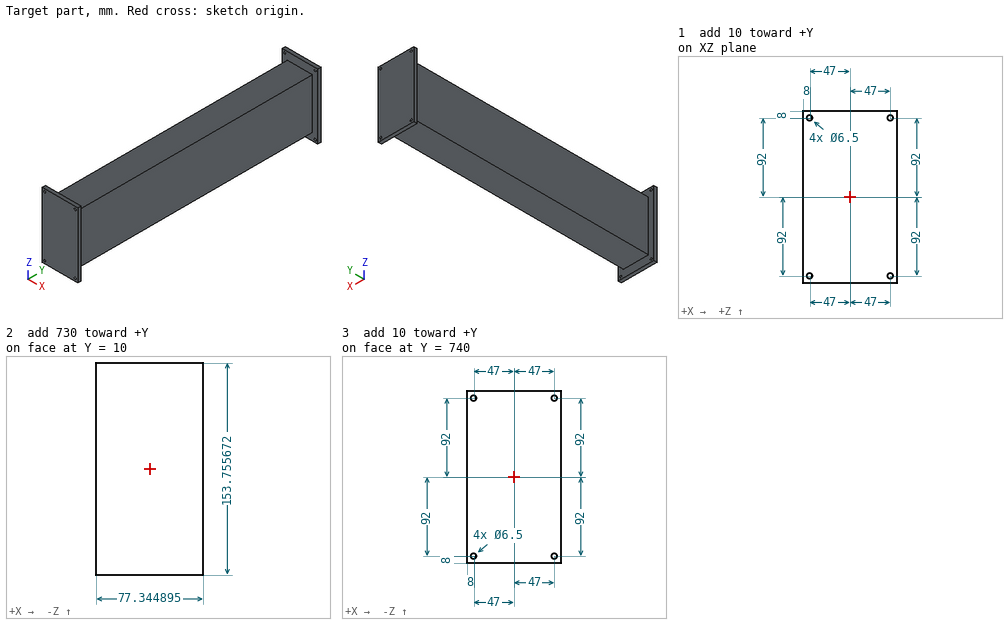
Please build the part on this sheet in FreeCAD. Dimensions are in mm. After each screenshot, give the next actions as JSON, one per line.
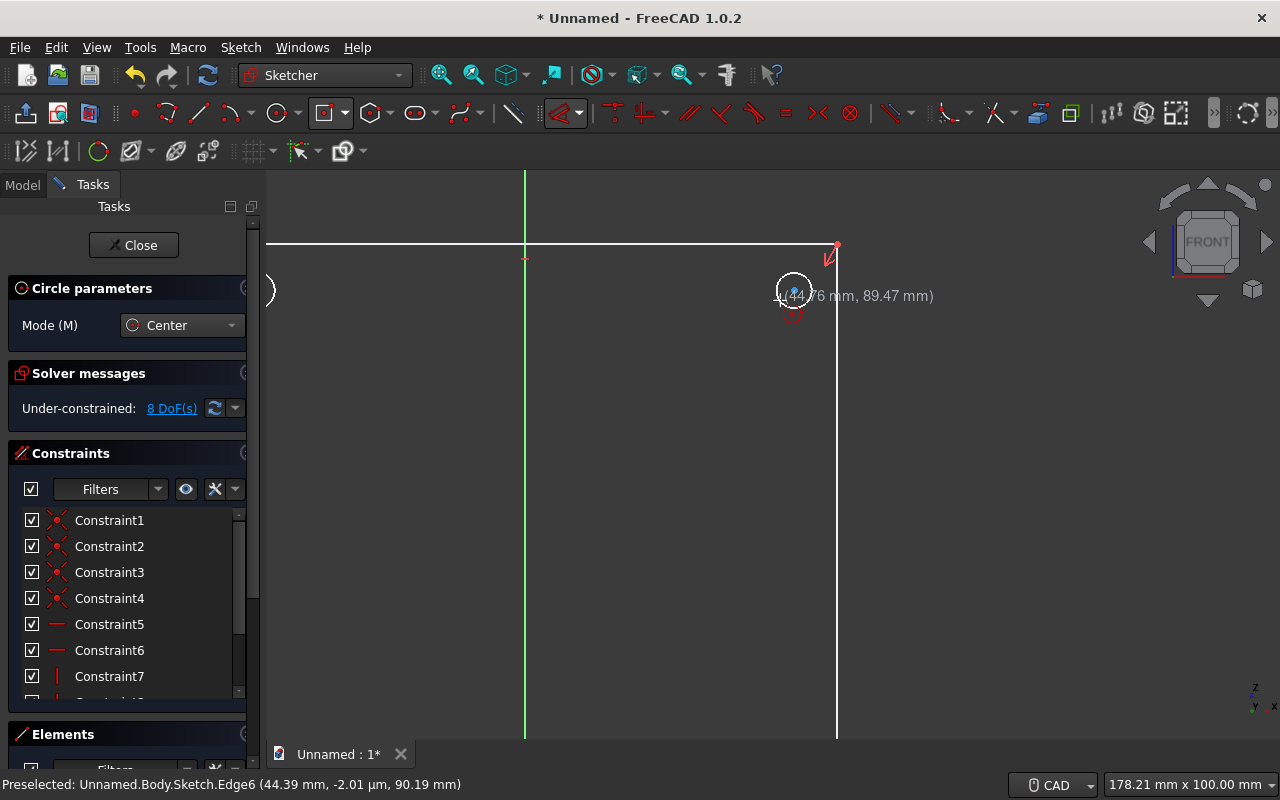
{"action": "scroll", "coordinate": [782, 301], "scroll_direction": "down", "scroll_amount": 6}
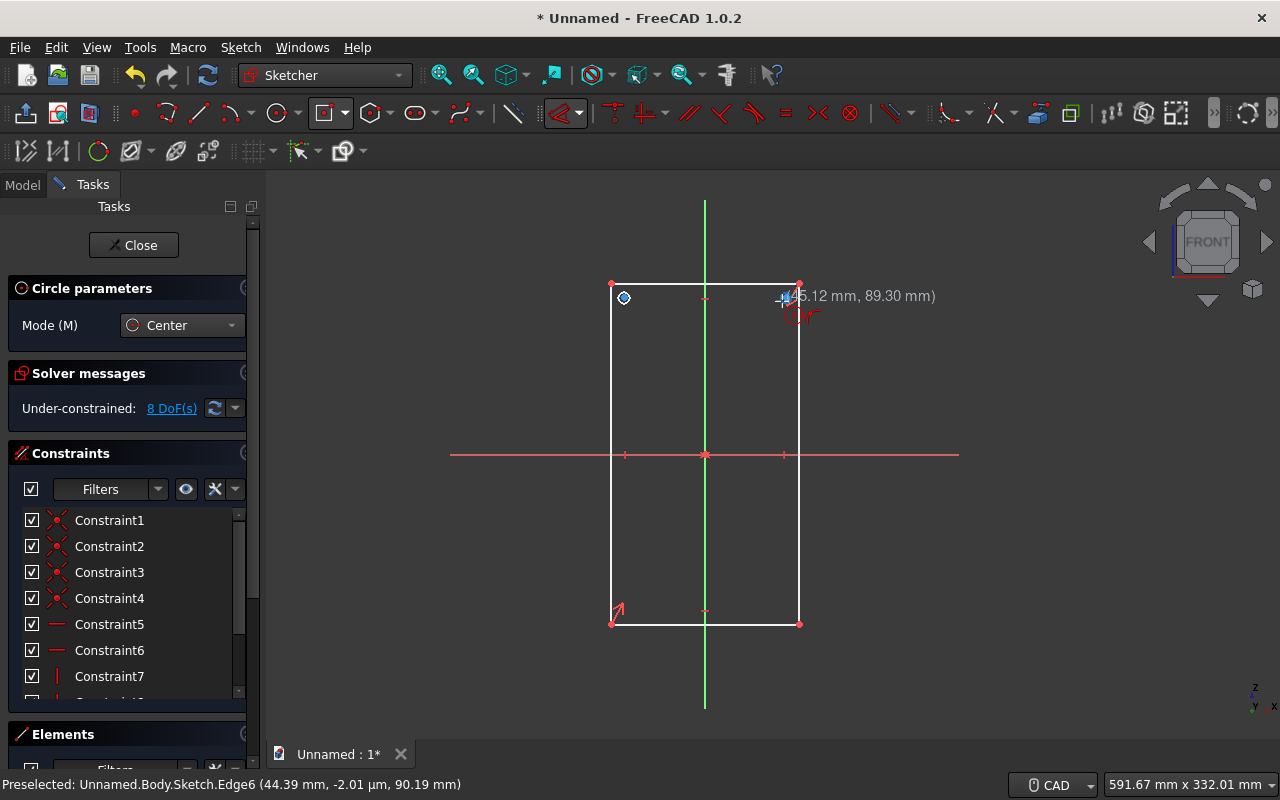
{"action": "scroll", "coordinate": [624, 612], "scroll_direction": "up", "scroll_amount": 8}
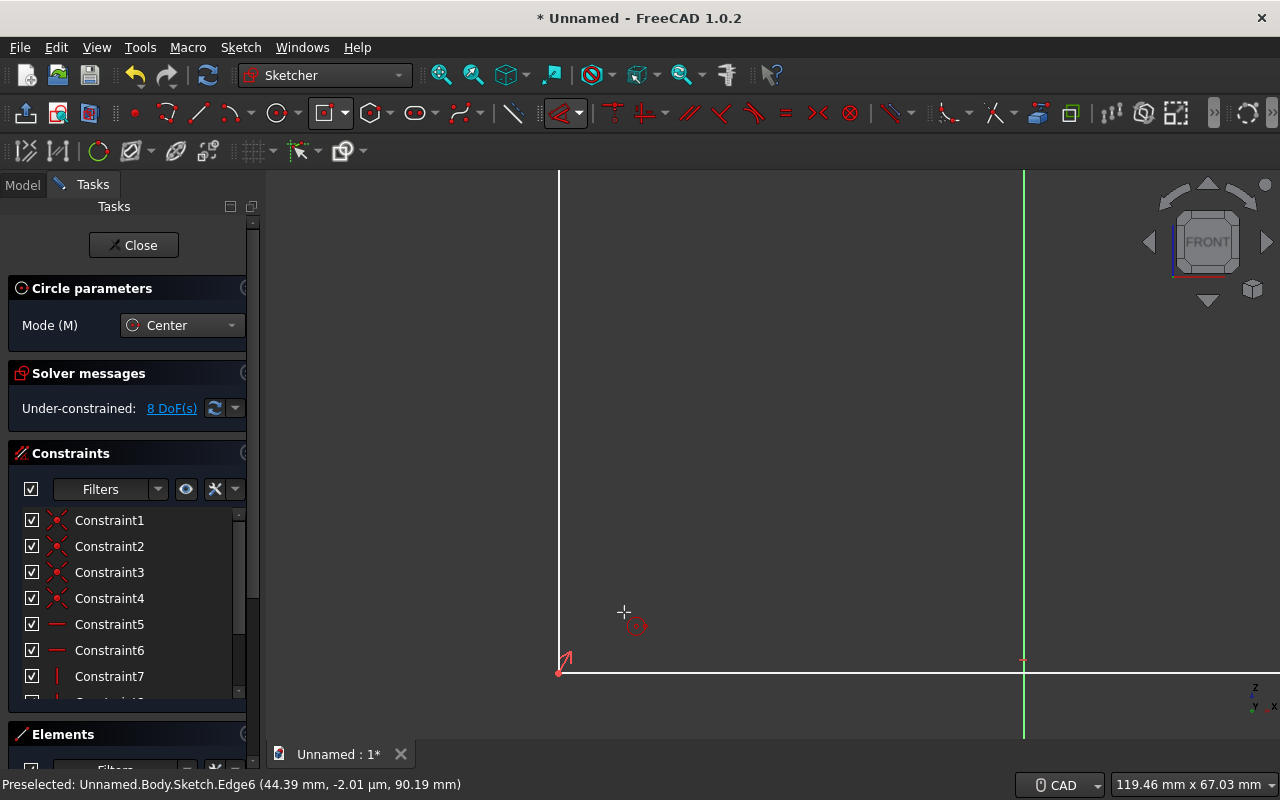
{"action": "scroll", "coordinate": [624, 613], "scroll_direction": "down", "scroll_amount": 8}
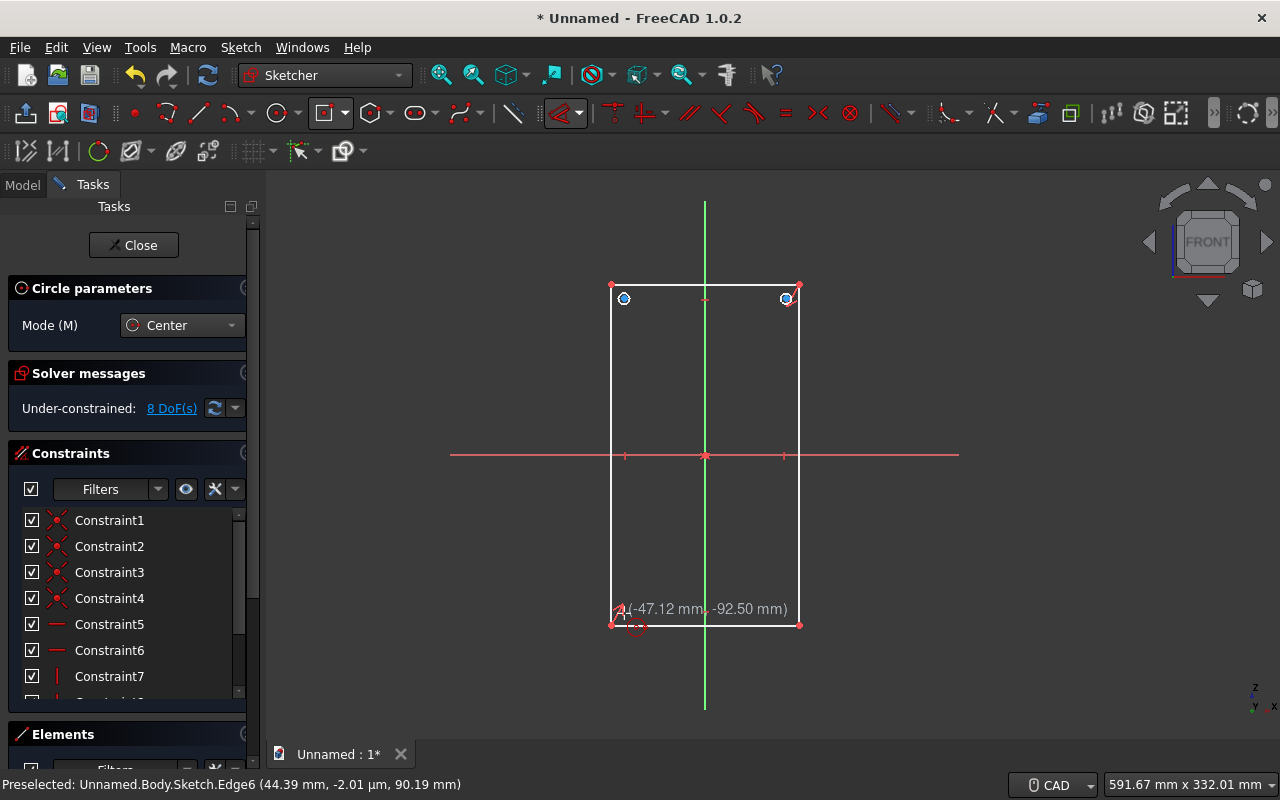
{"action": "left_click", "coordinate": [624, 613]}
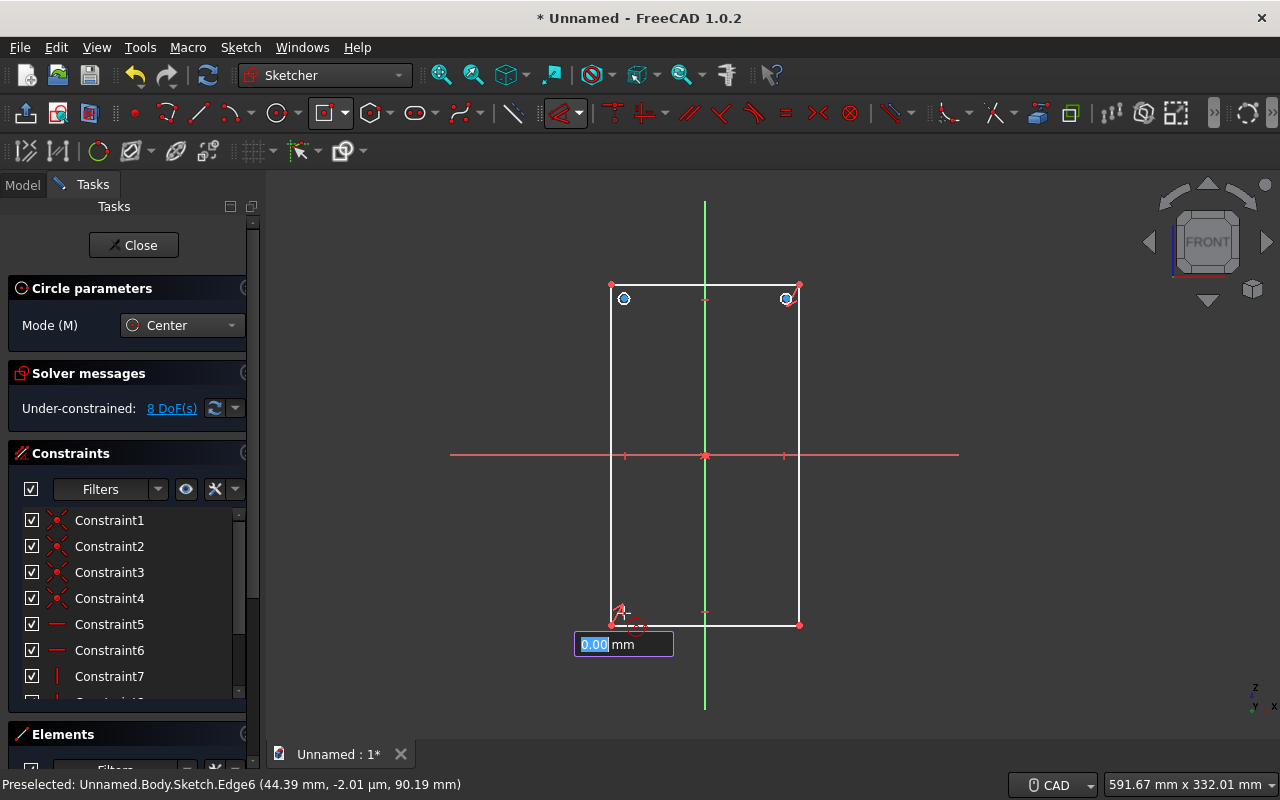
{"action": "scroll", "coordinate": [628, 609], "scroll_direction": "up", "scroll_amount": 6}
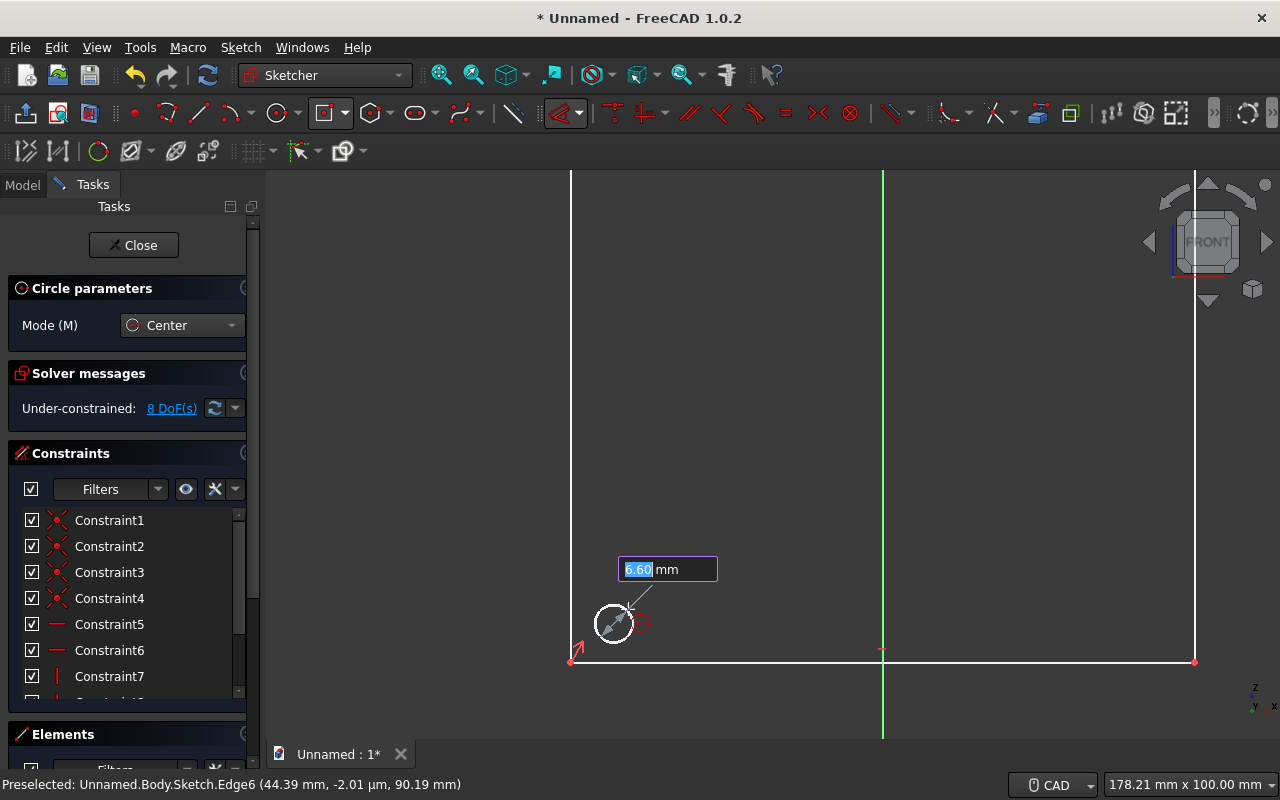
{"action": "left_click", "coordinate": [629, 607]}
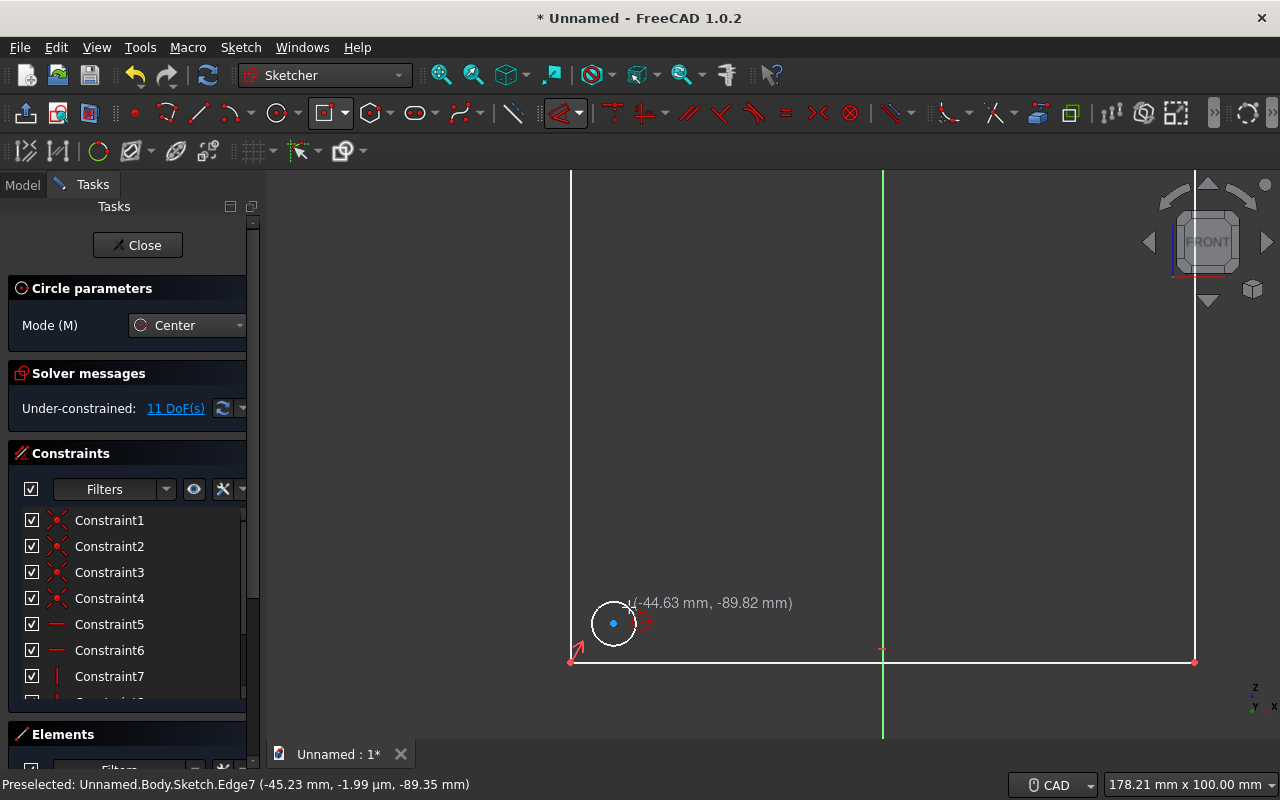
{"action": "scroll", "coordinate": [628, 609], "scroll_direction": "down", "scroll_amount": 6}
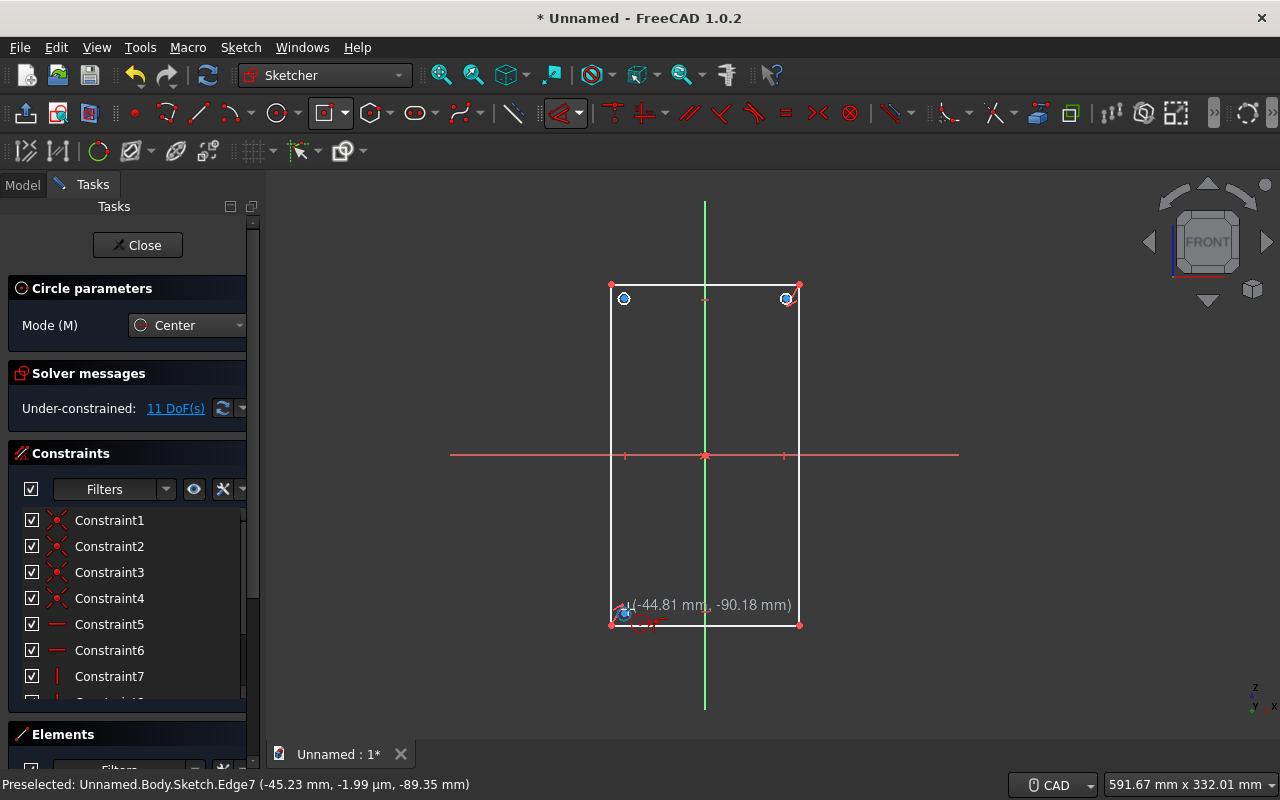
{"action": "scroll", "coordinate": [786, 613], "scroll_direction": "up", "scroll_amount": 8}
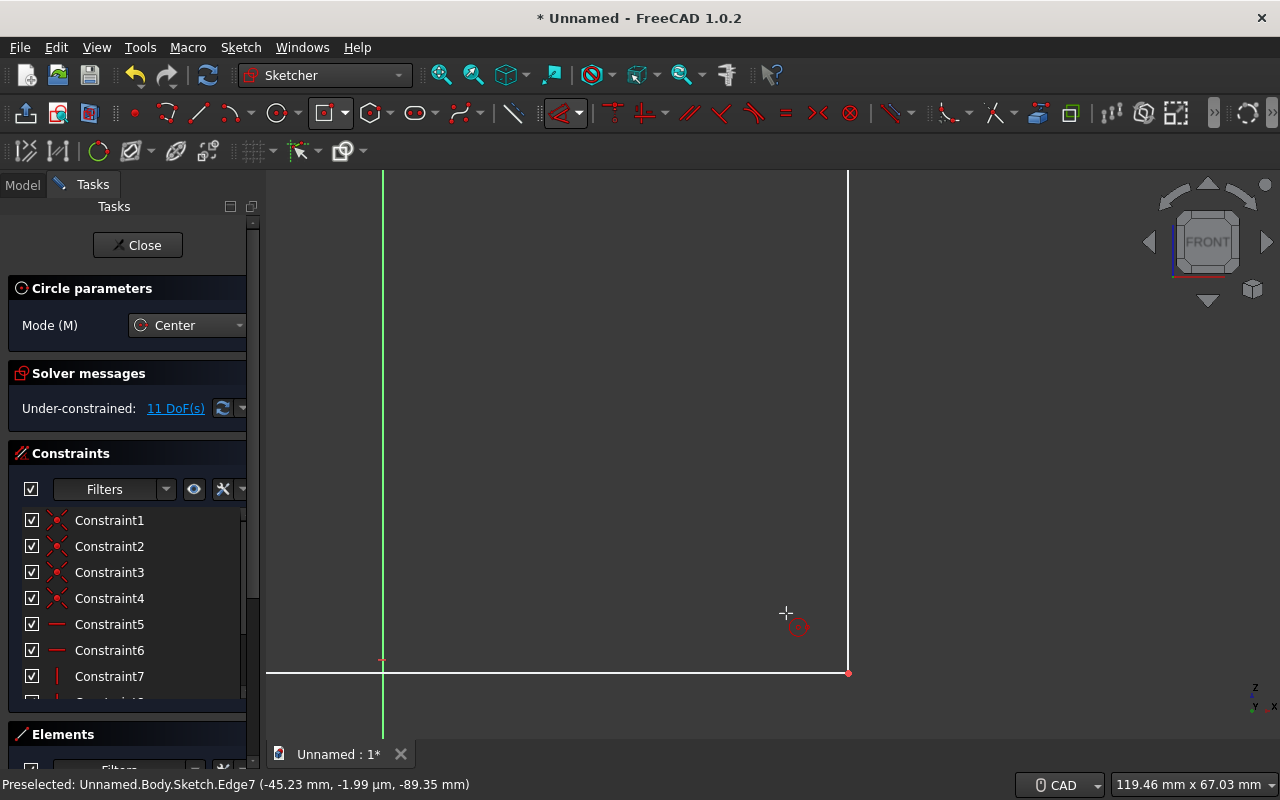
{"action": "scroll", "coordinate": [786, 613], "scroll_direction": "down", "scroll_amount": 8}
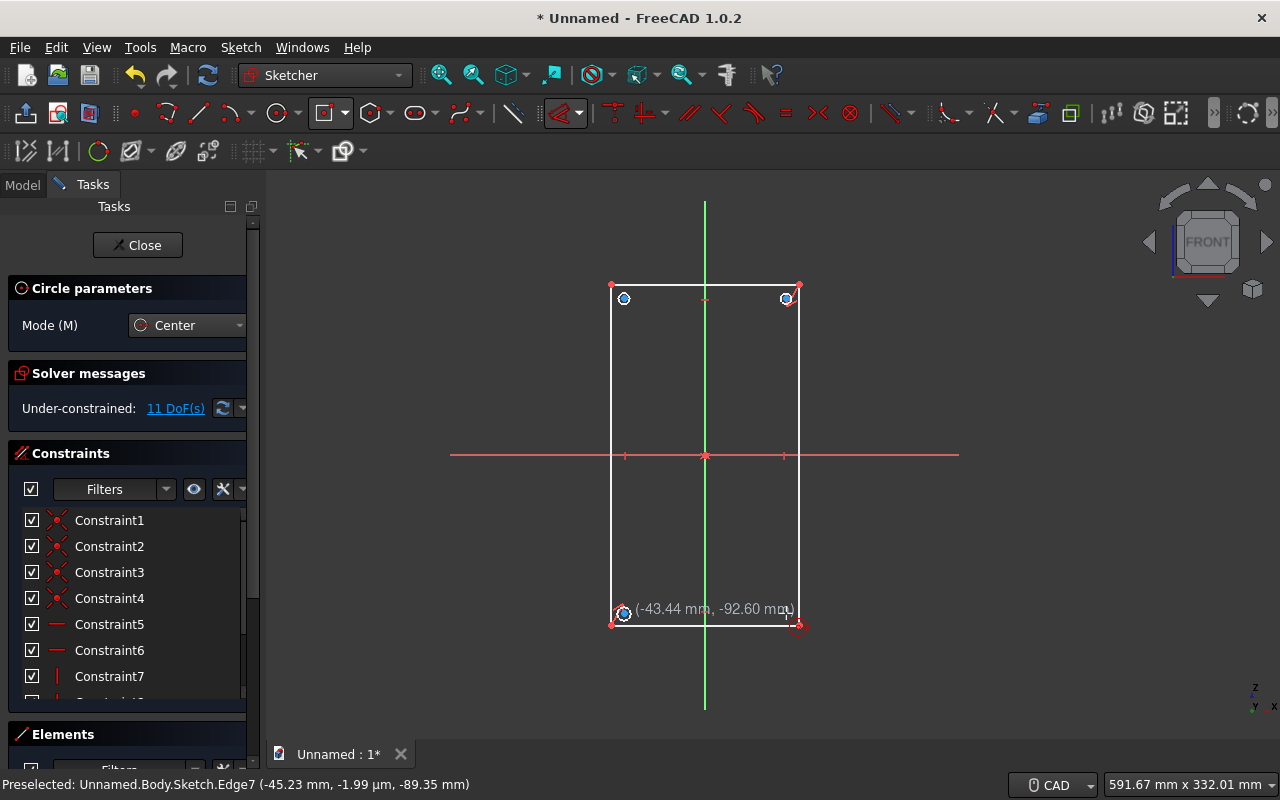
{"action": "left_click", "coordinate": [786, 613]}